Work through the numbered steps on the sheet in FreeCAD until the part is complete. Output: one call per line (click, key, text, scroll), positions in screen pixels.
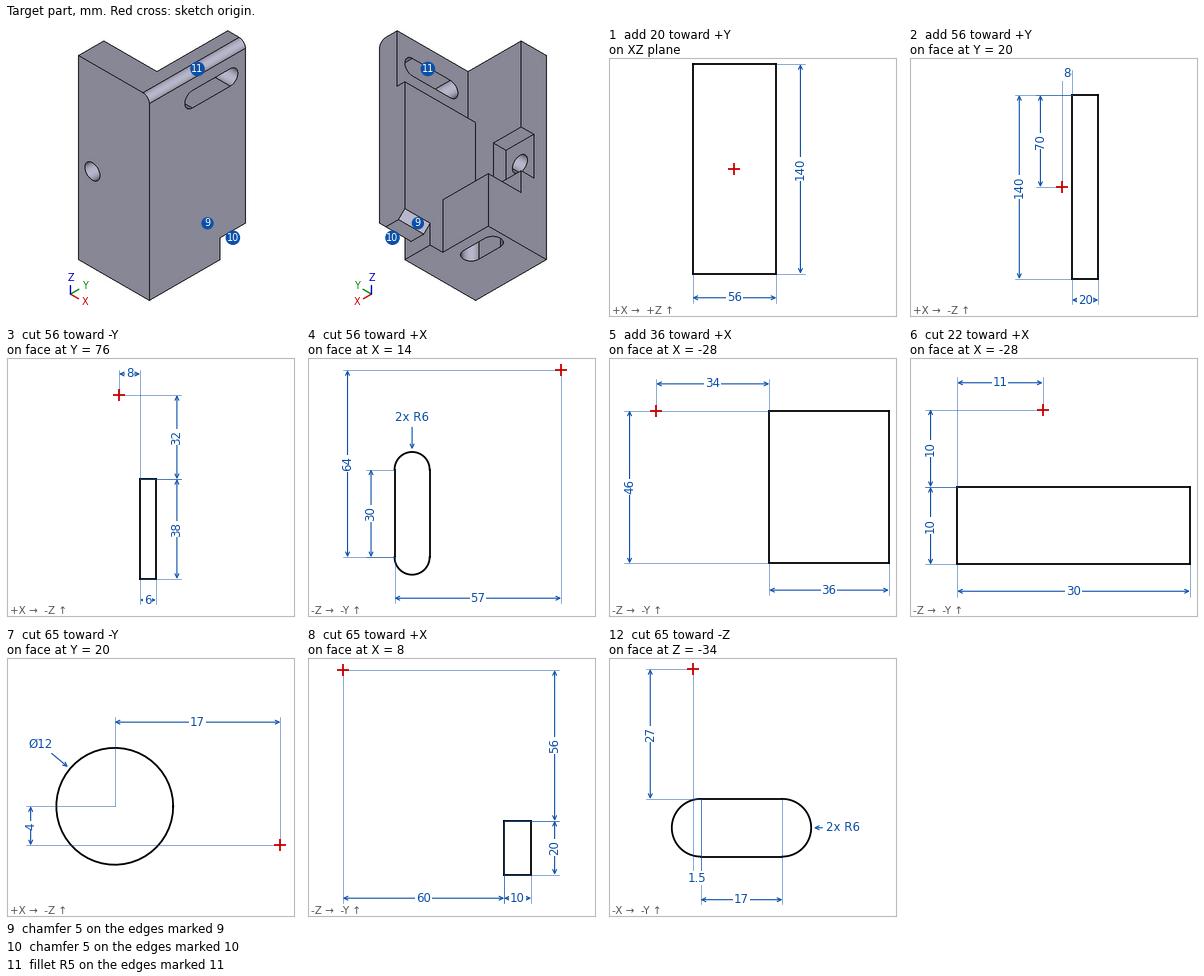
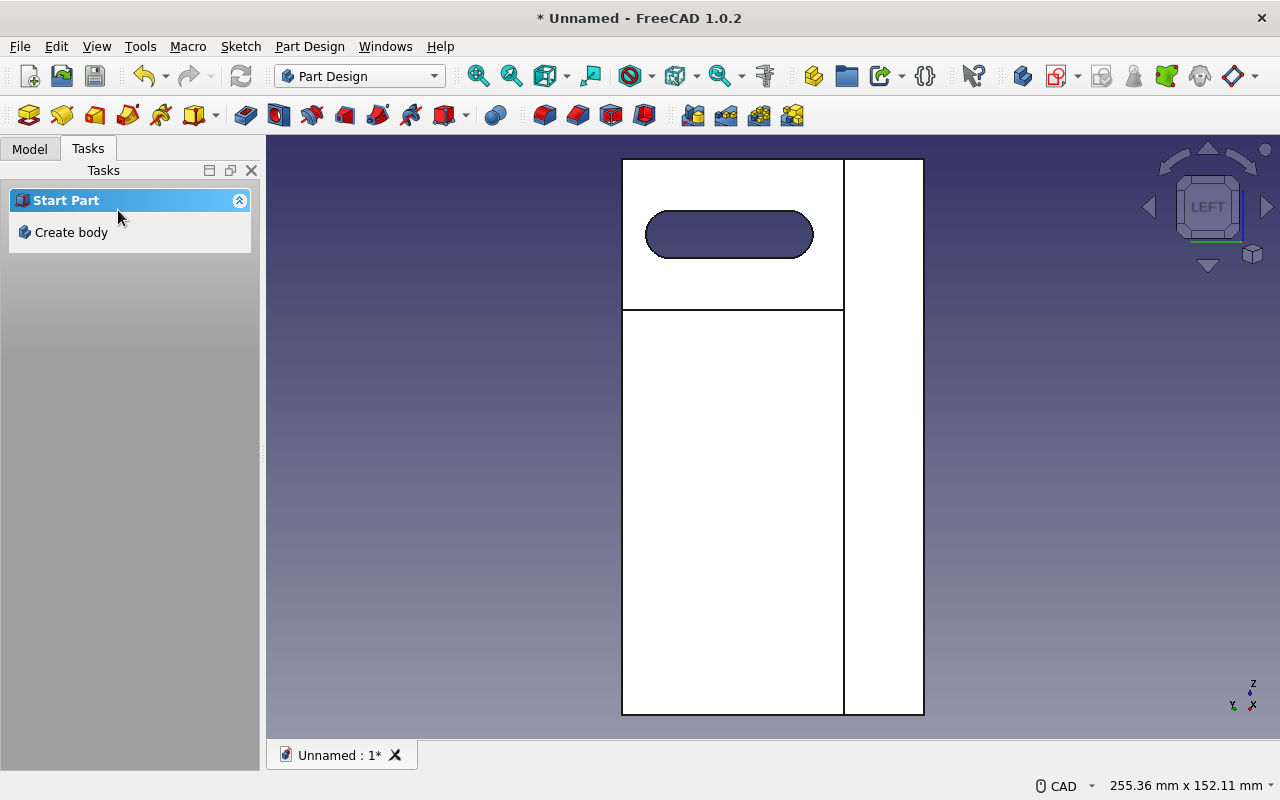
click(884, 436)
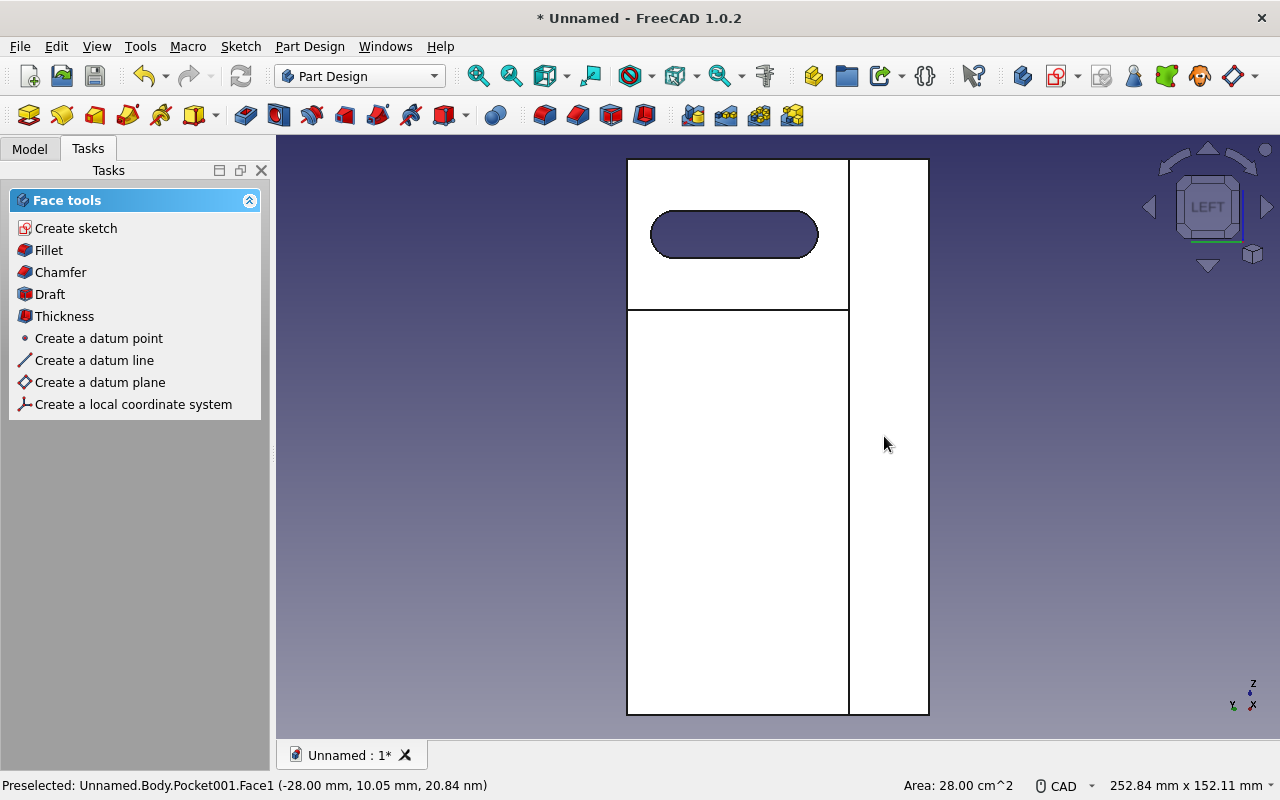
click(1056, 76)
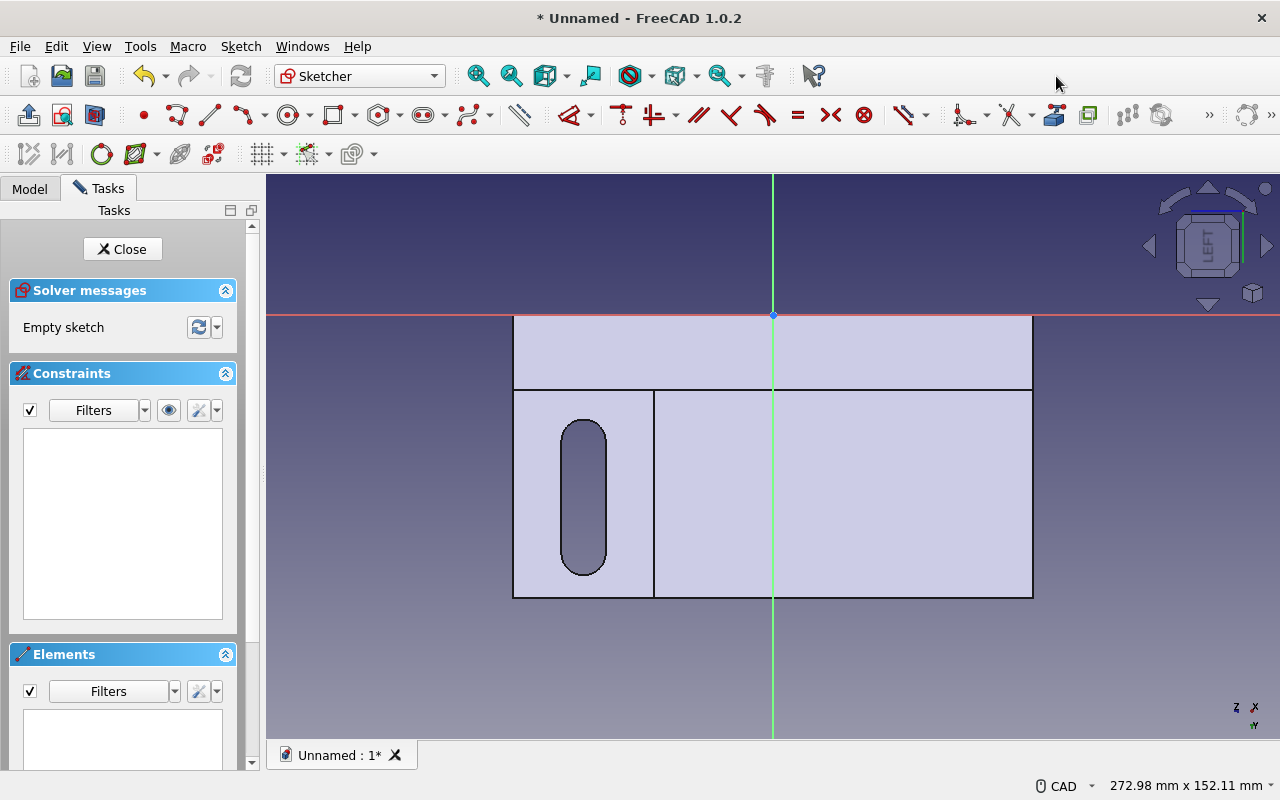
scroll(1065, 355, up, 4)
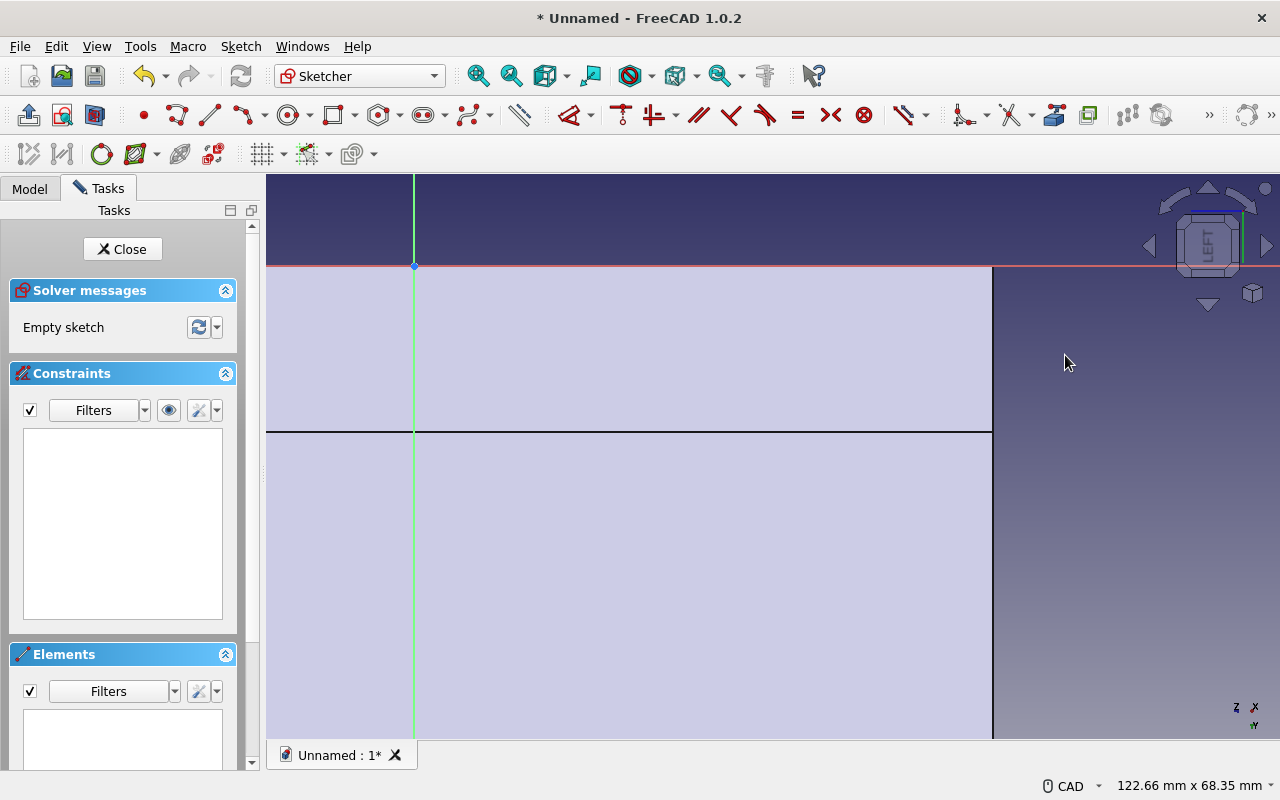
click(332, 116)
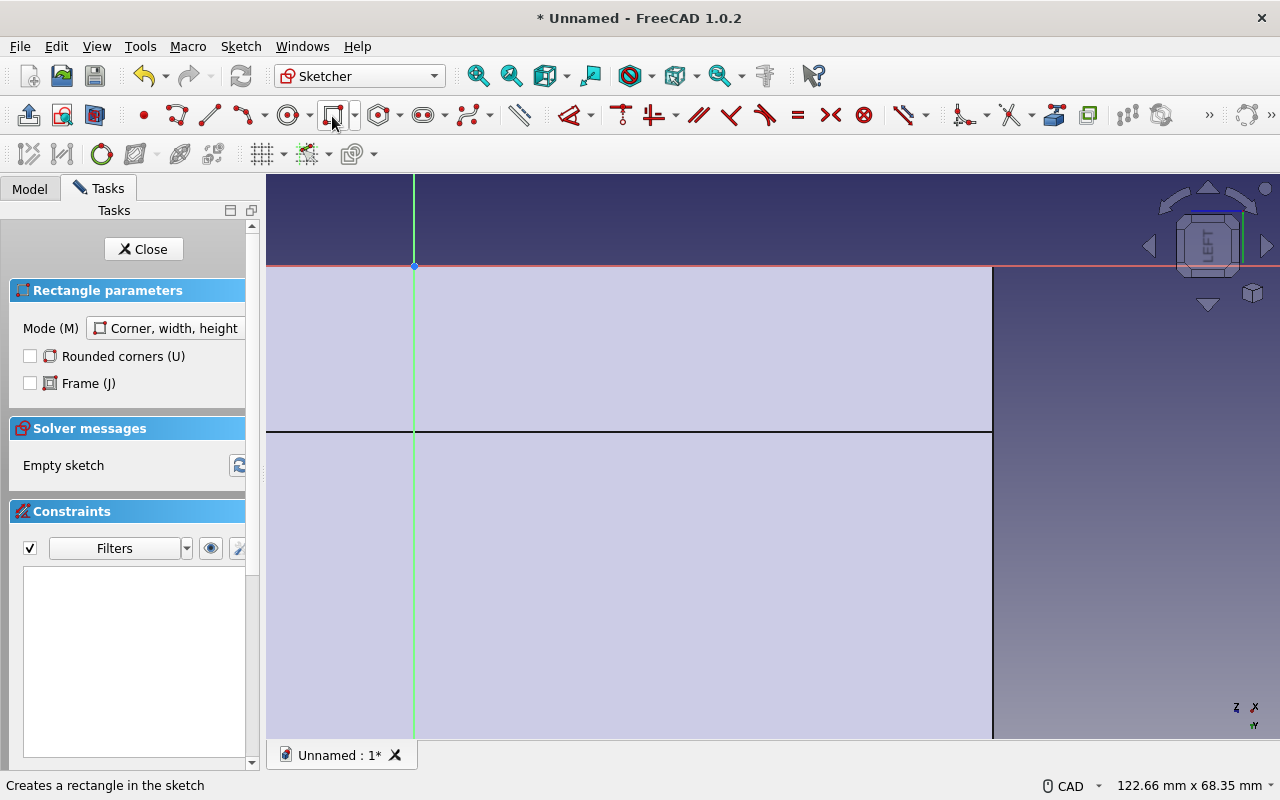
click(695, 266)
click(993, 647)
key(Escape)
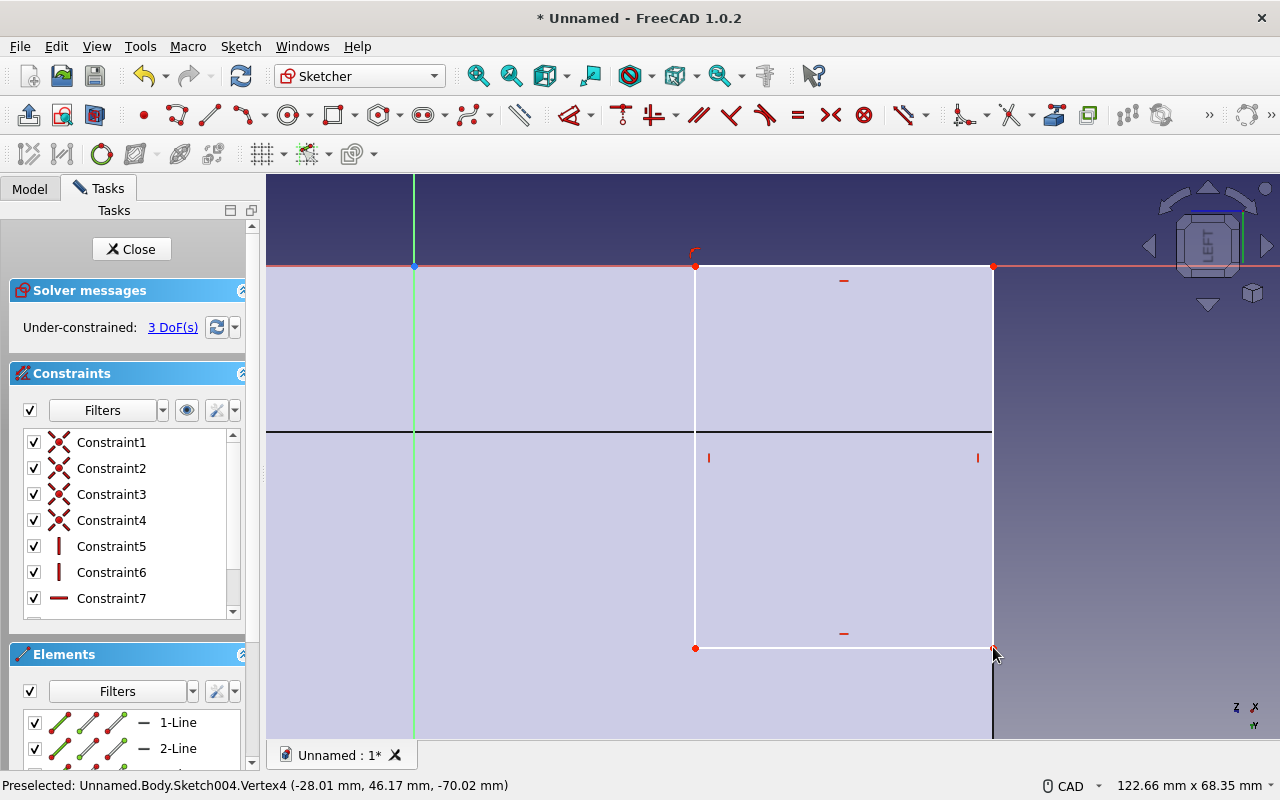
click(568, 116)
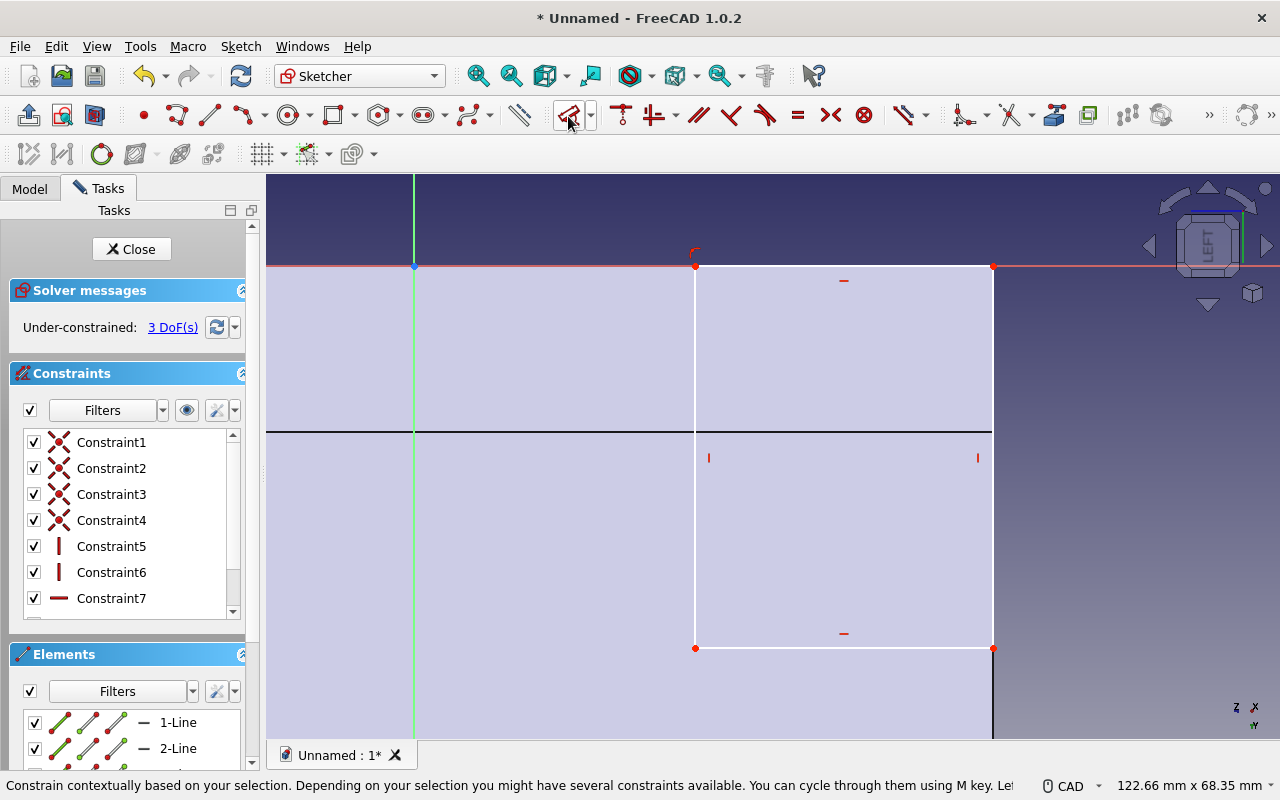
click(695, 381)
click(661, 457)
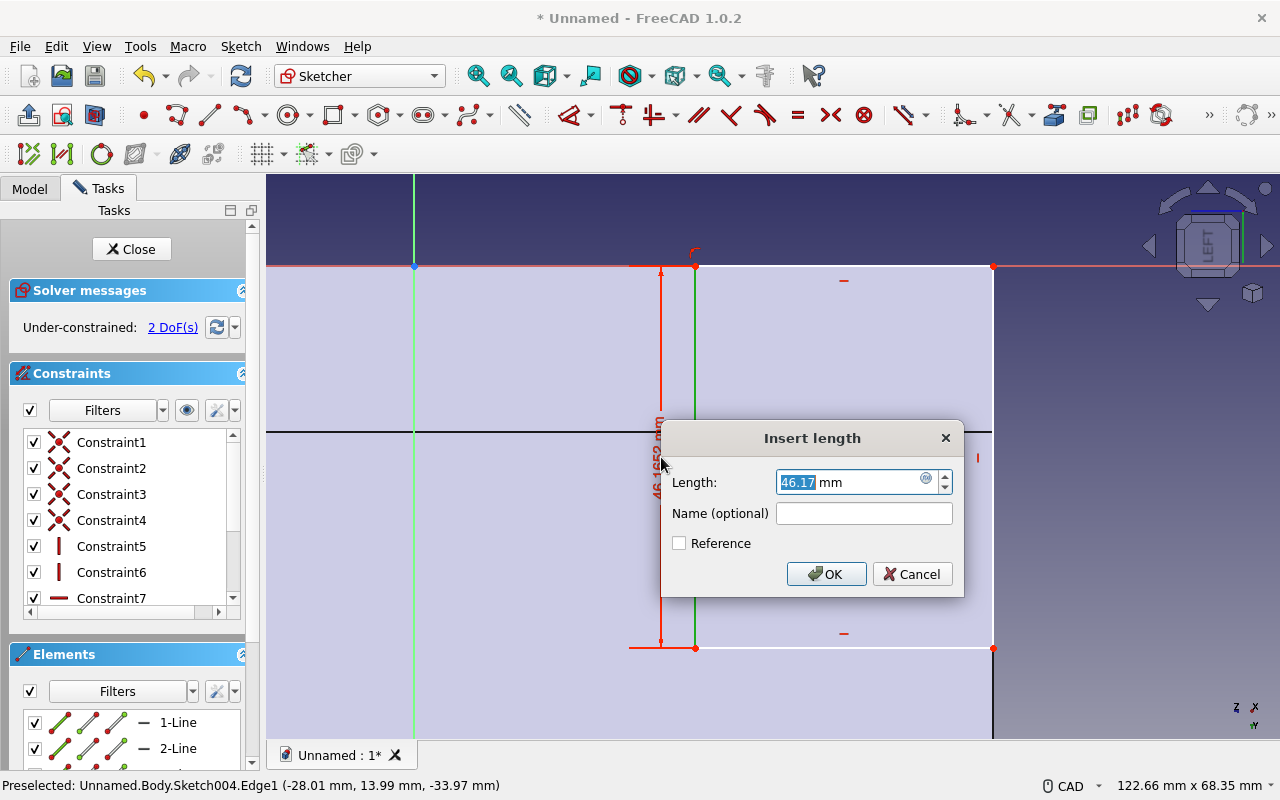
text(46)
key(Return)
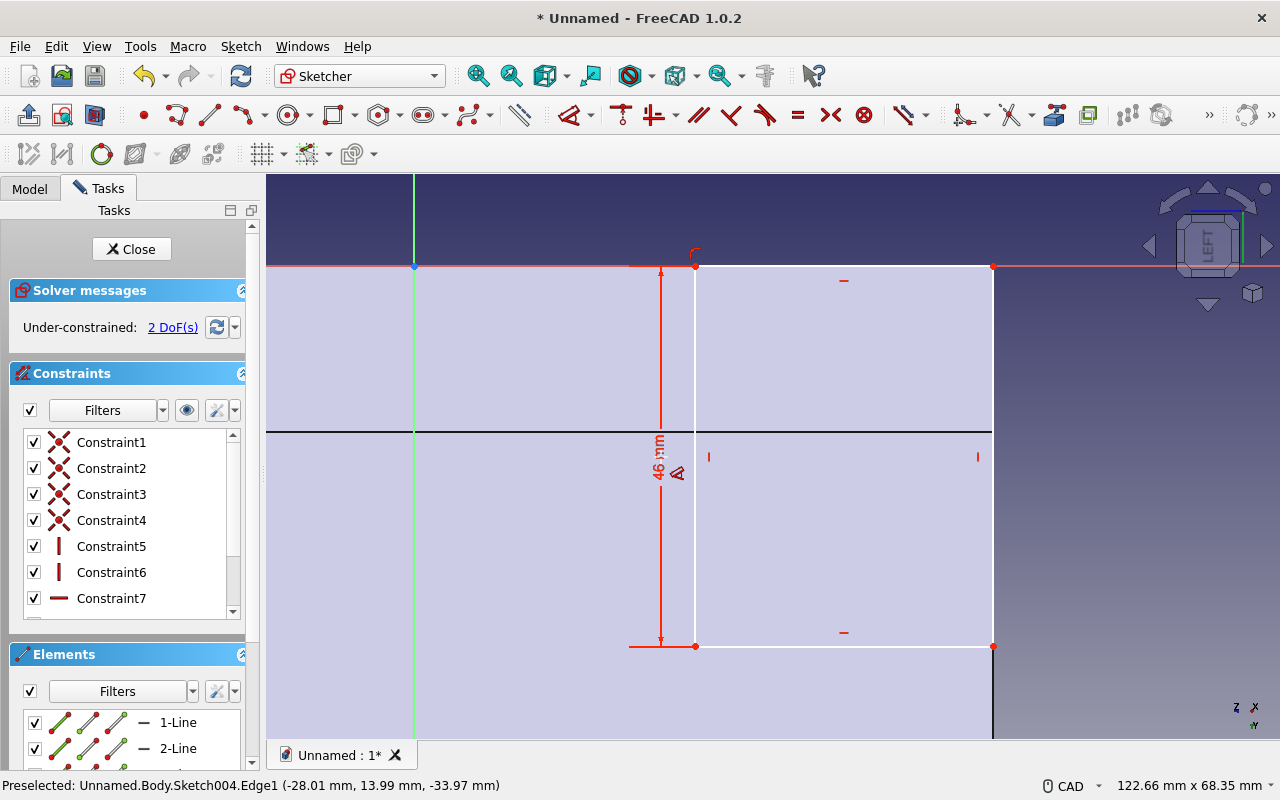
click(784, 647)
click(844, 681)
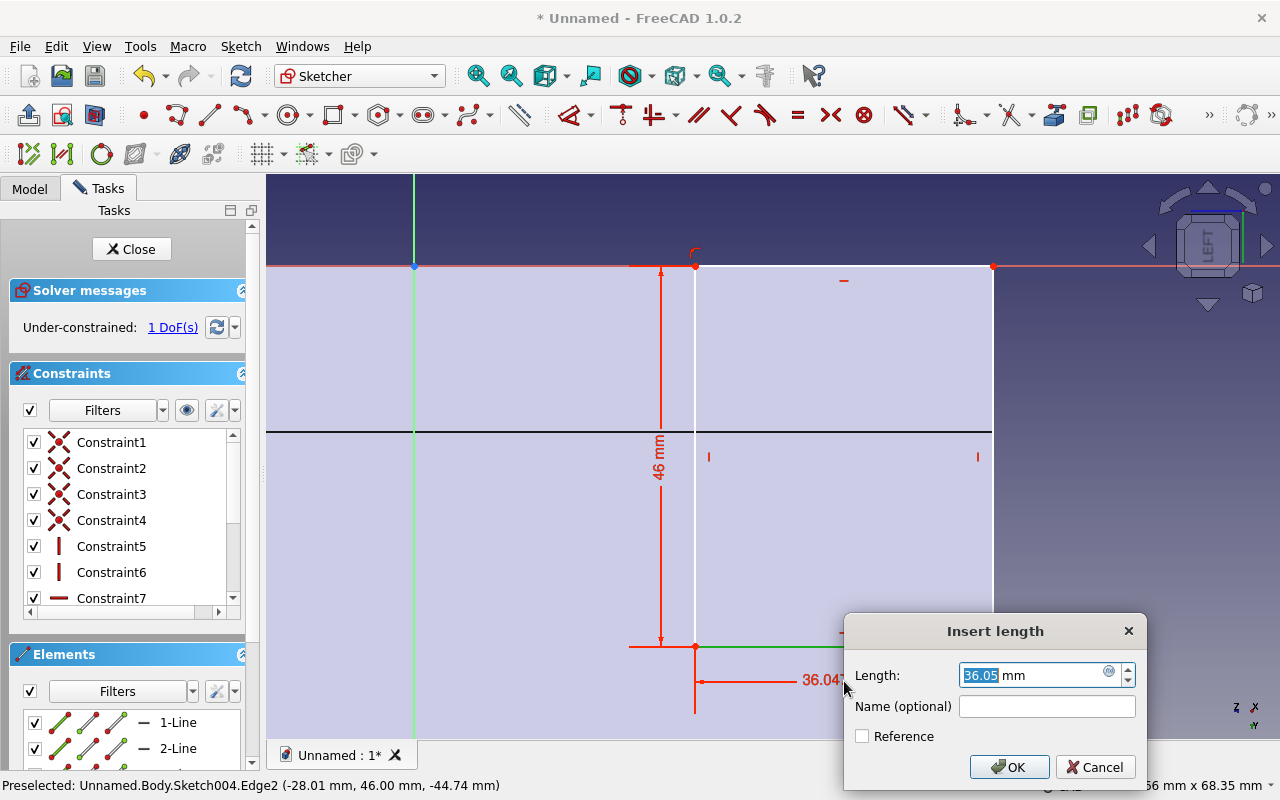
text(36)
key(Return)